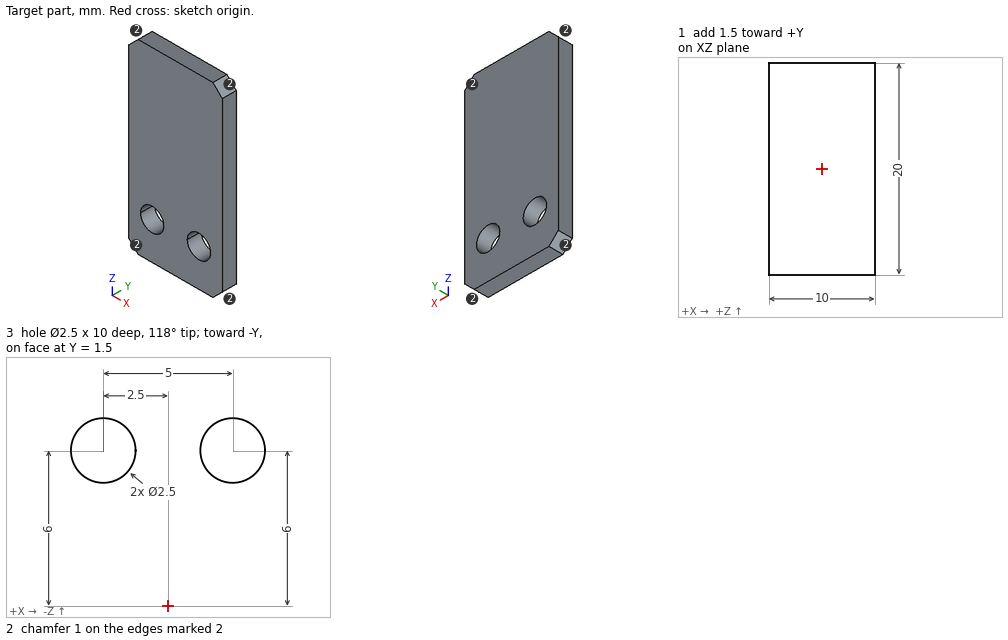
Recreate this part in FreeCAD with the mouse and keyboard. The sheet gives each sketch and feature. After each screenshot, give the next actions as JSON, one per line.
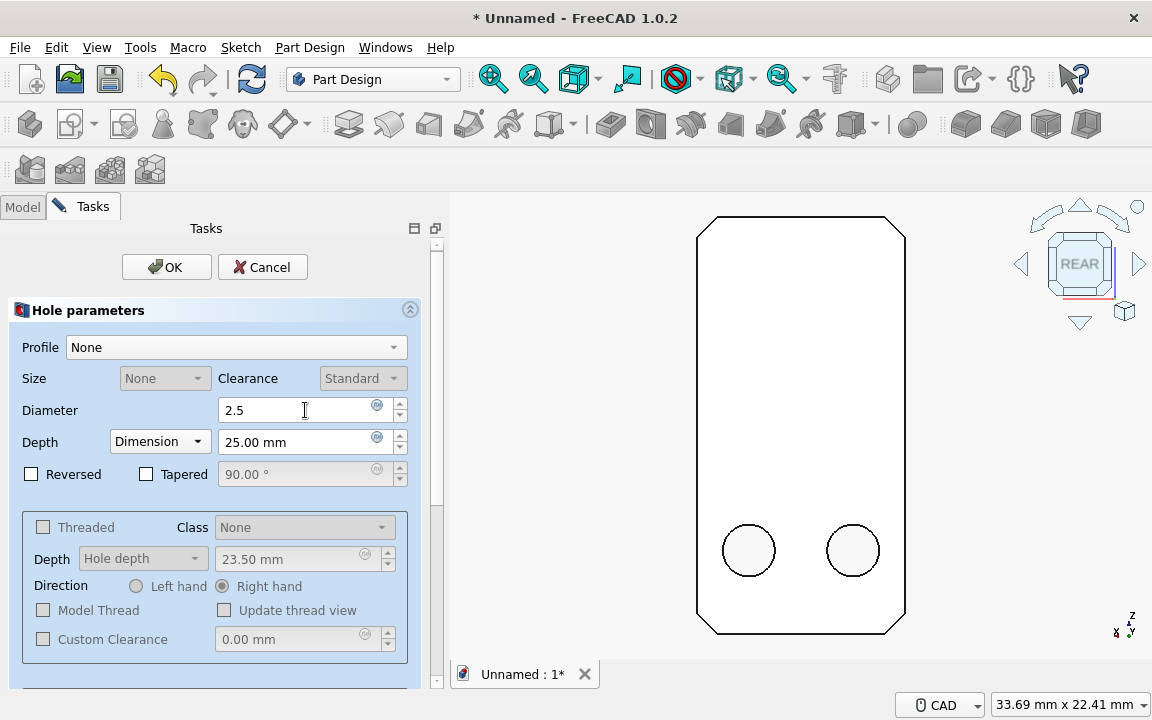
{"action": "triple_click", "coordinate": [305, 442]}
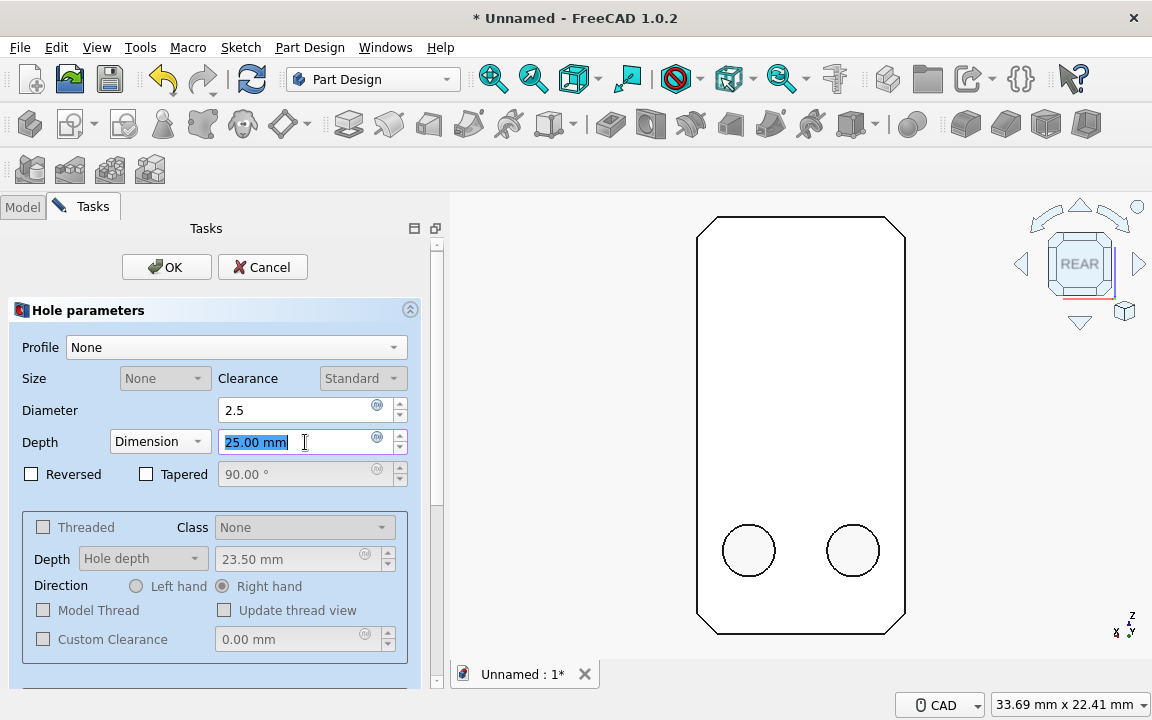
{"action": "type", "text": "10"}
{"action": "key", "text": "Tab"}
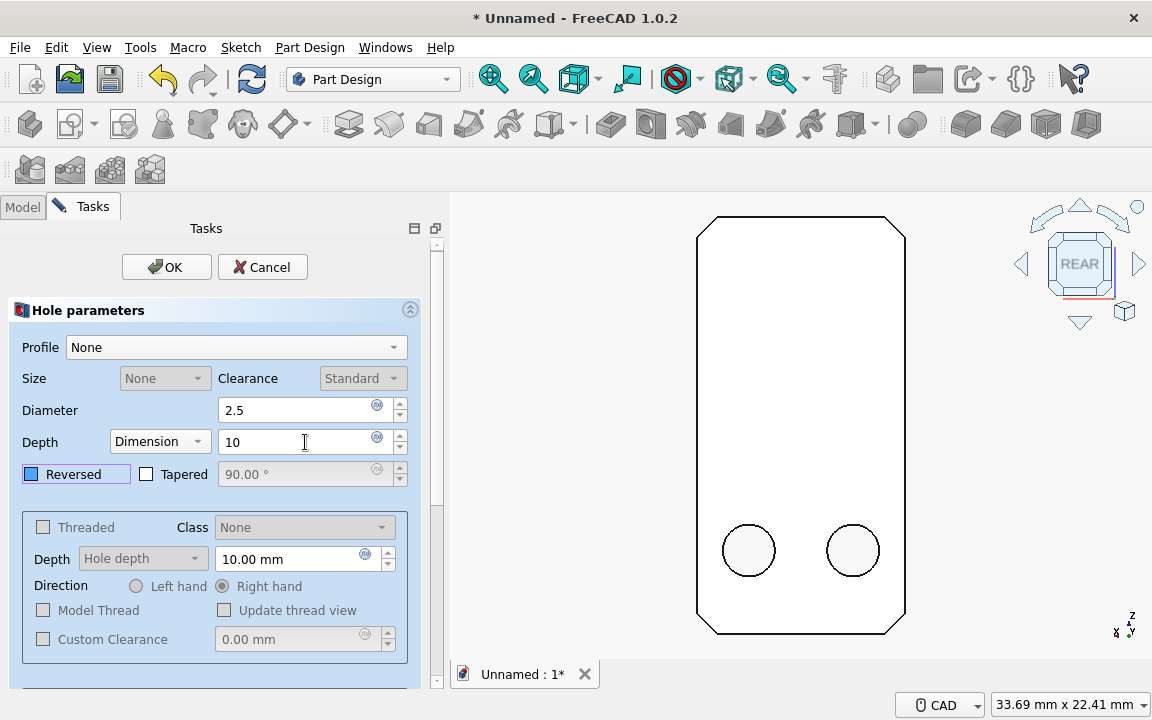
{"action": "left_click", "coordinate": [167, 267]}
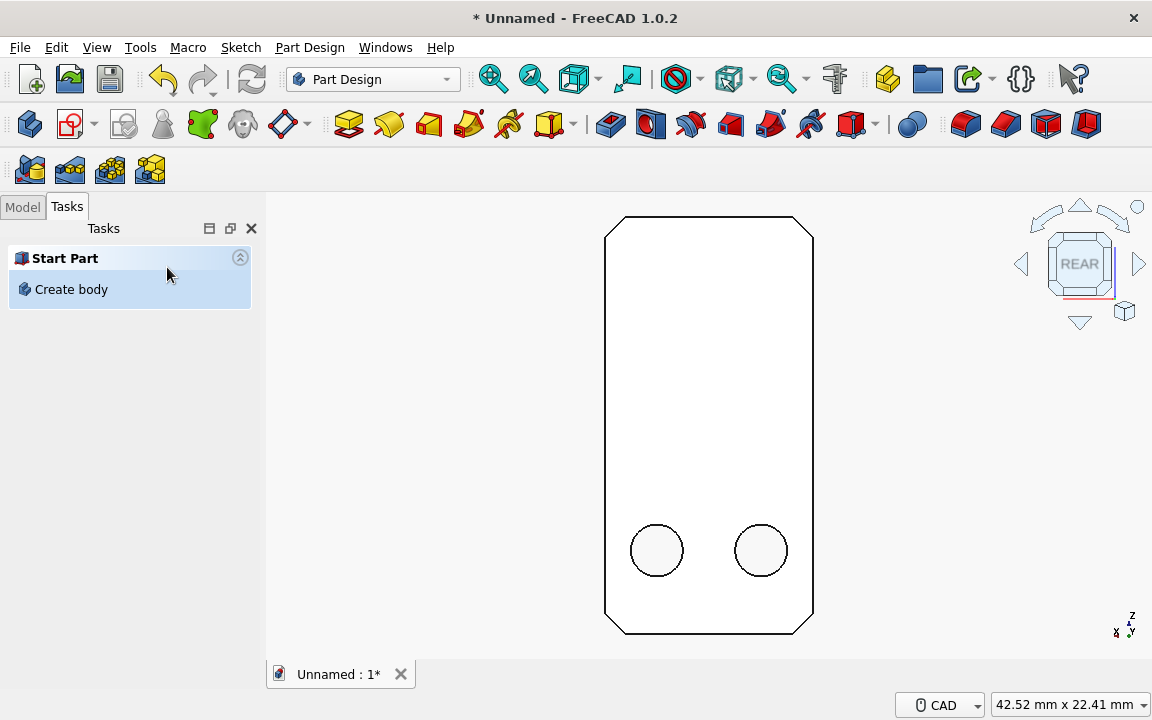
{"action": "key", "text": "0"}